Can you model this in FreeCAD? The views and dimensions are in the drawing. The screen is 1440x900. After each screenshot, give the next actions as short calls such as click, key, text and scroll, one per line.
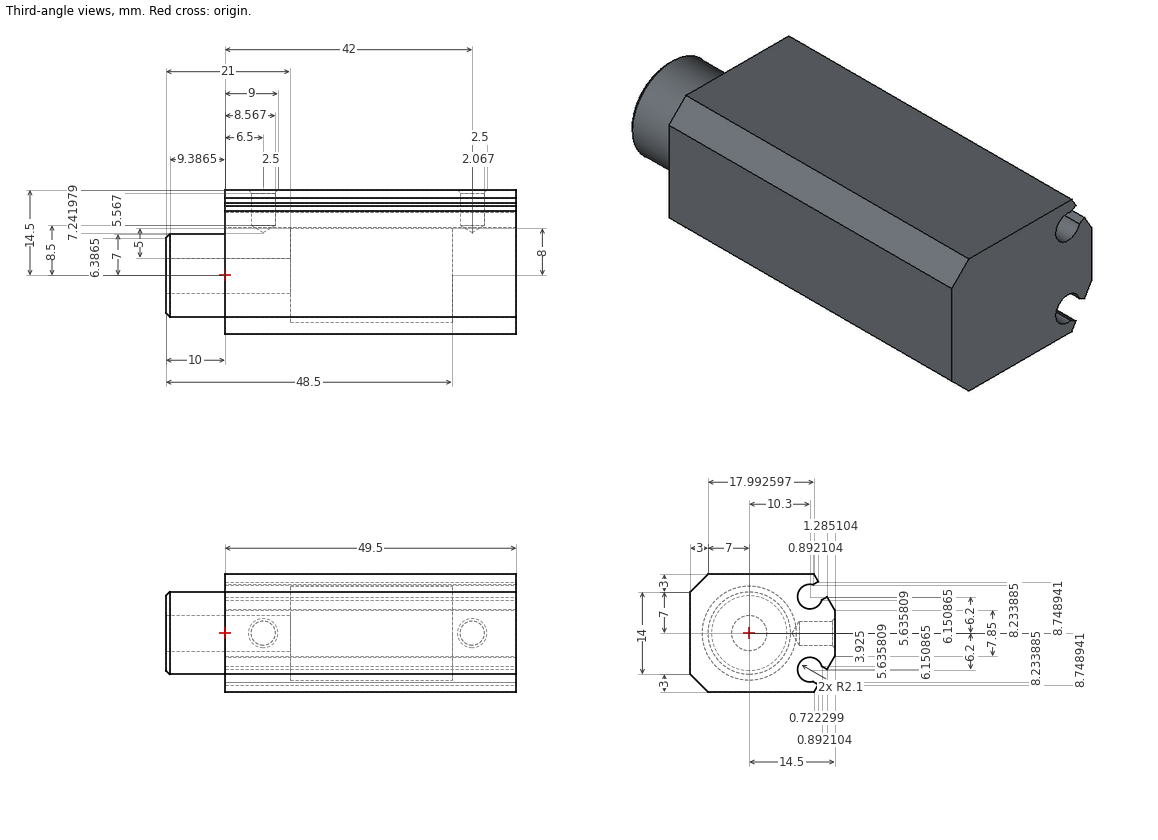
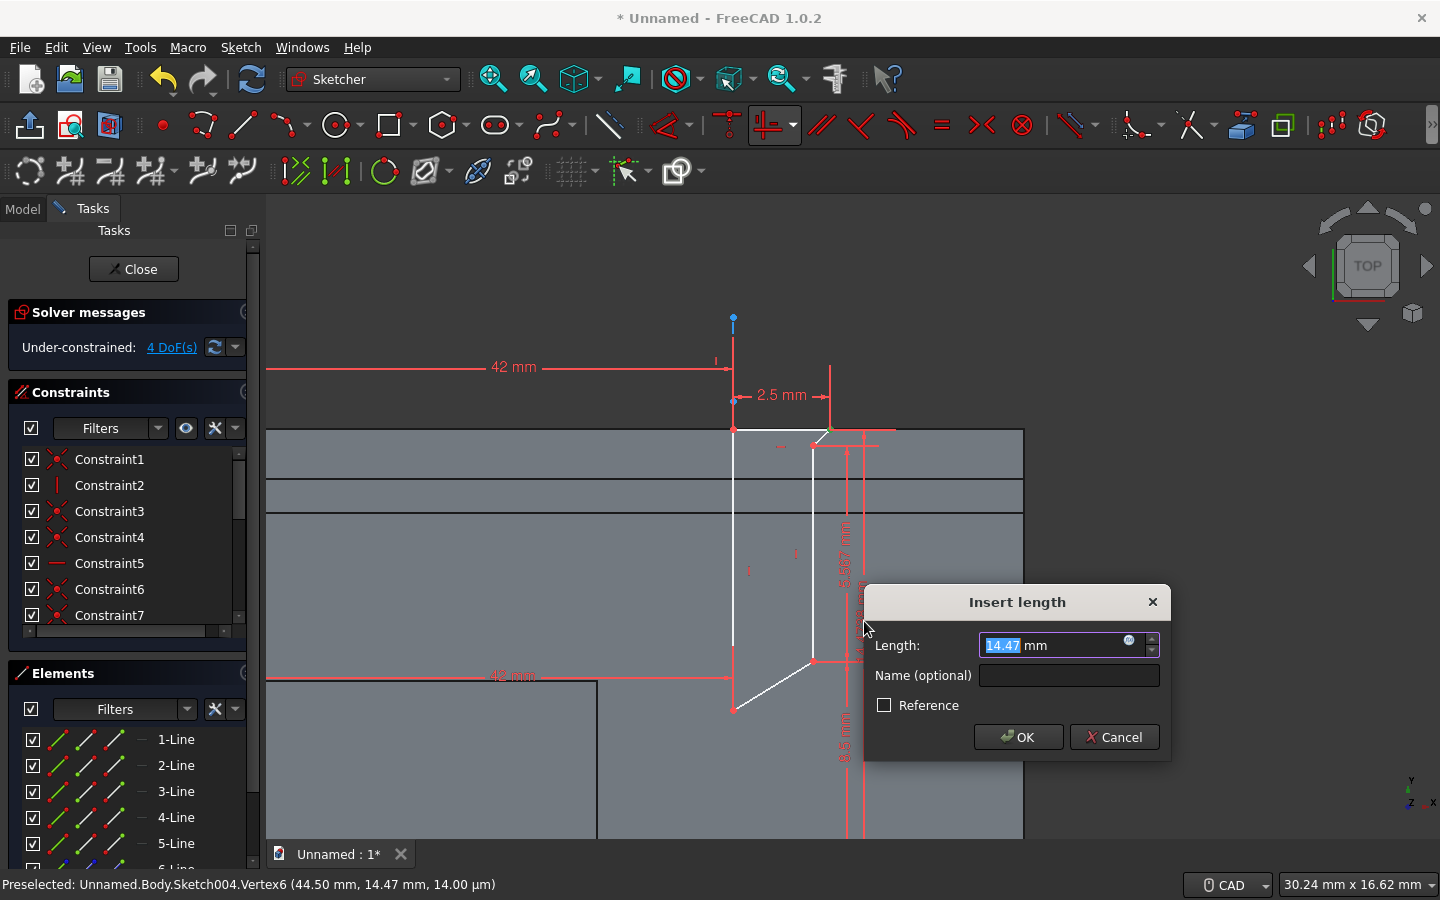
text(14.5)
key(Return)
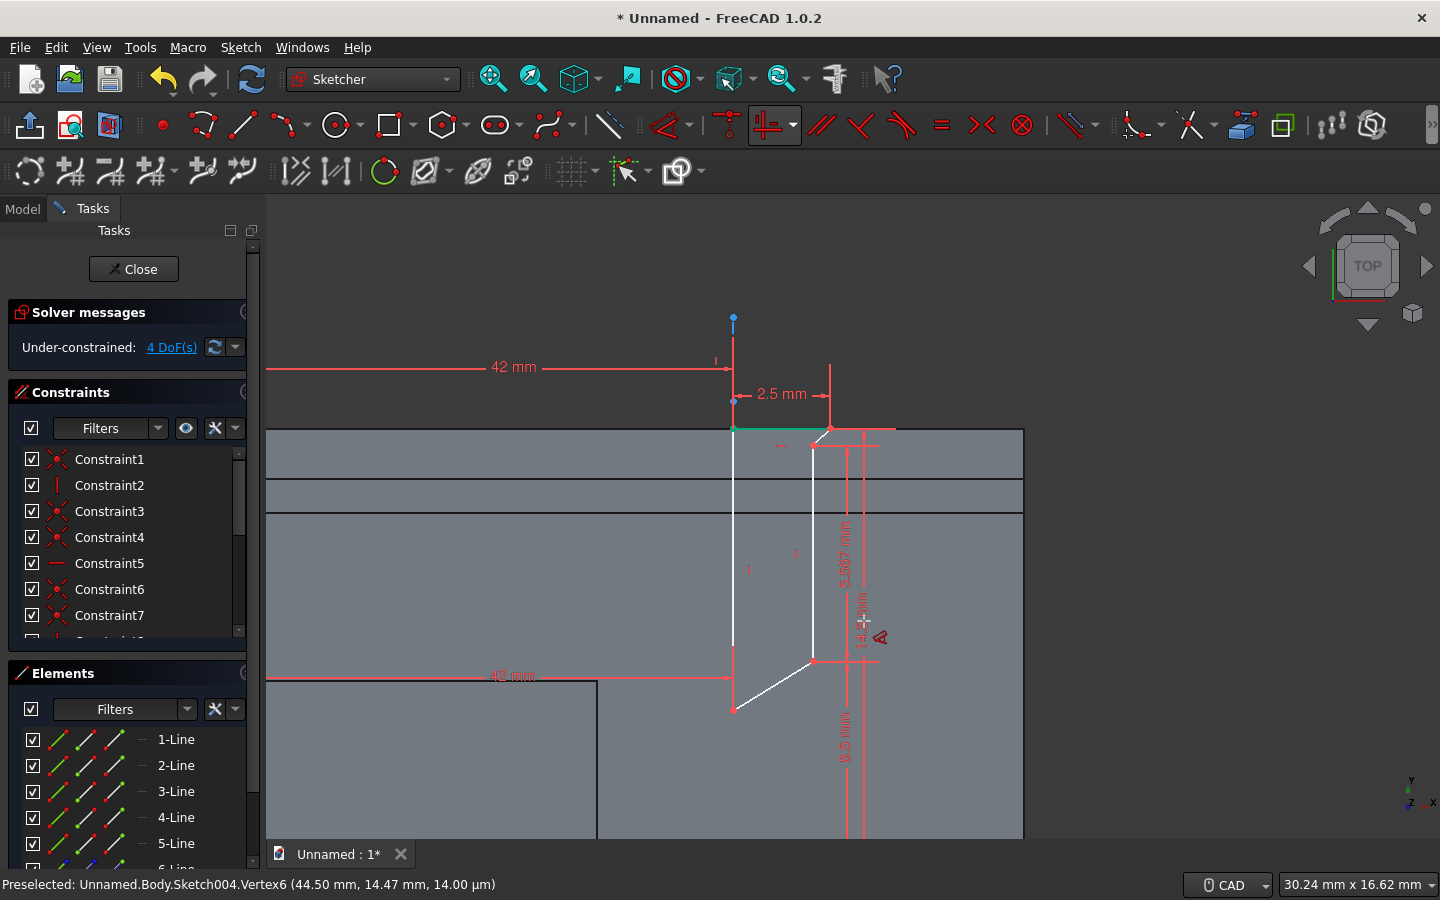
click(757, 696)
click(773, 745)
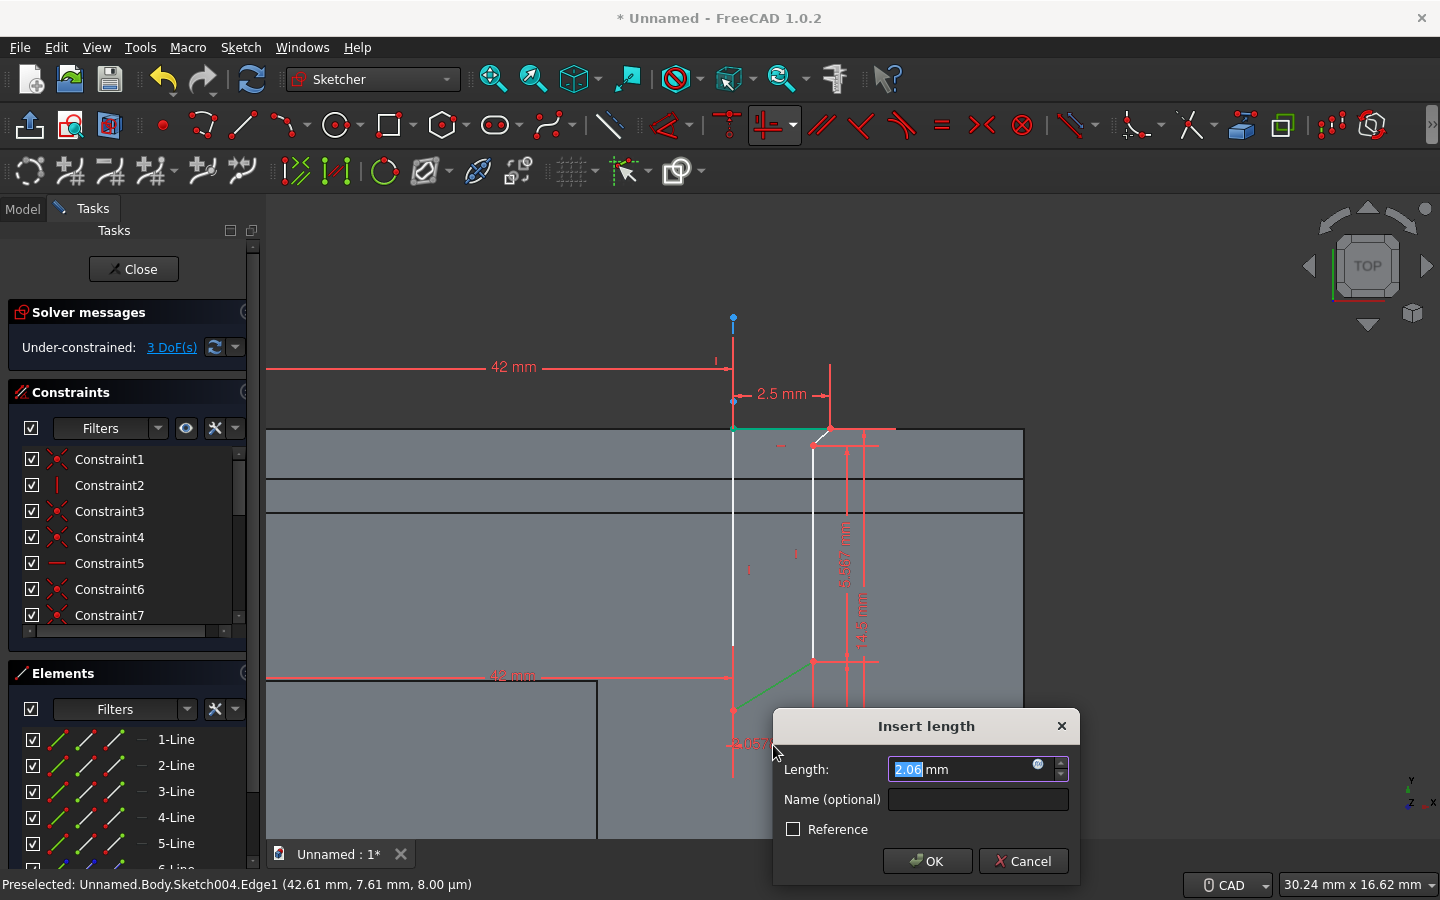
text(2.067)
key(Return)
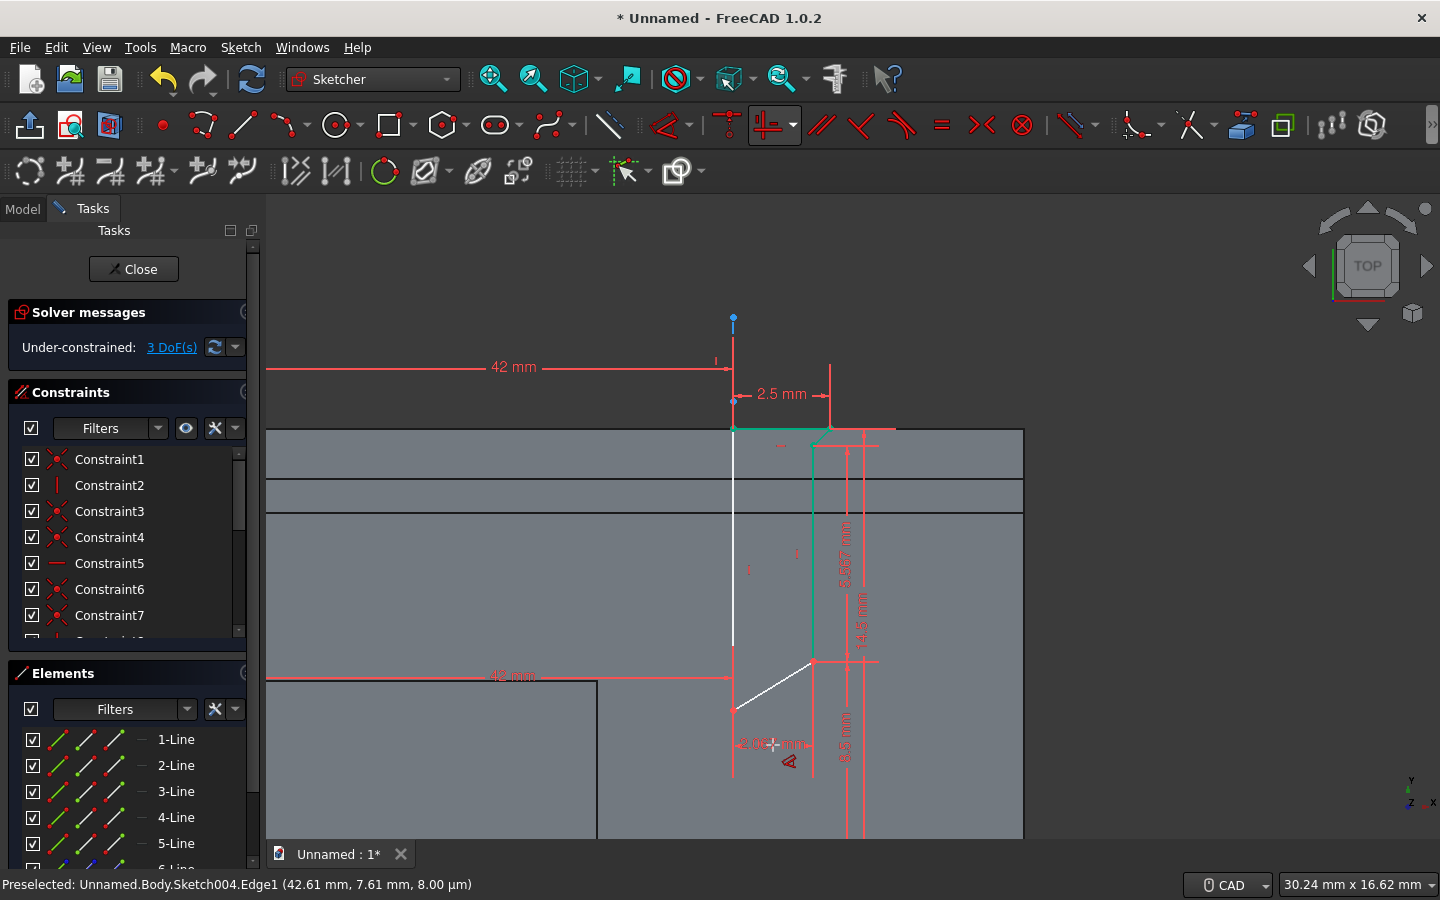
click(733, 514)
click(699, 570)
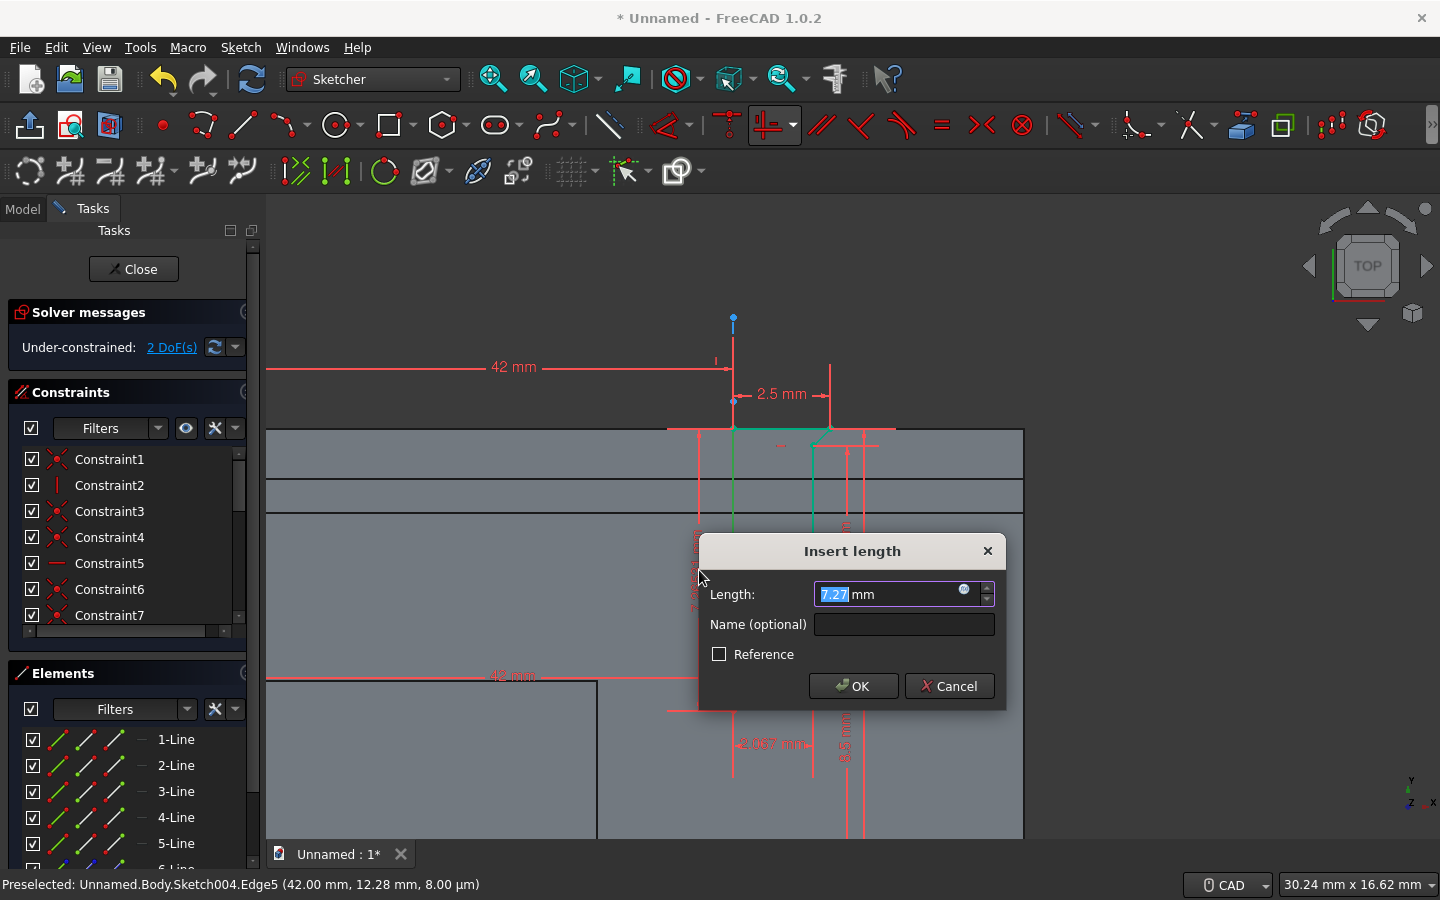
text(7.241979)
key(Return)
key(Escape)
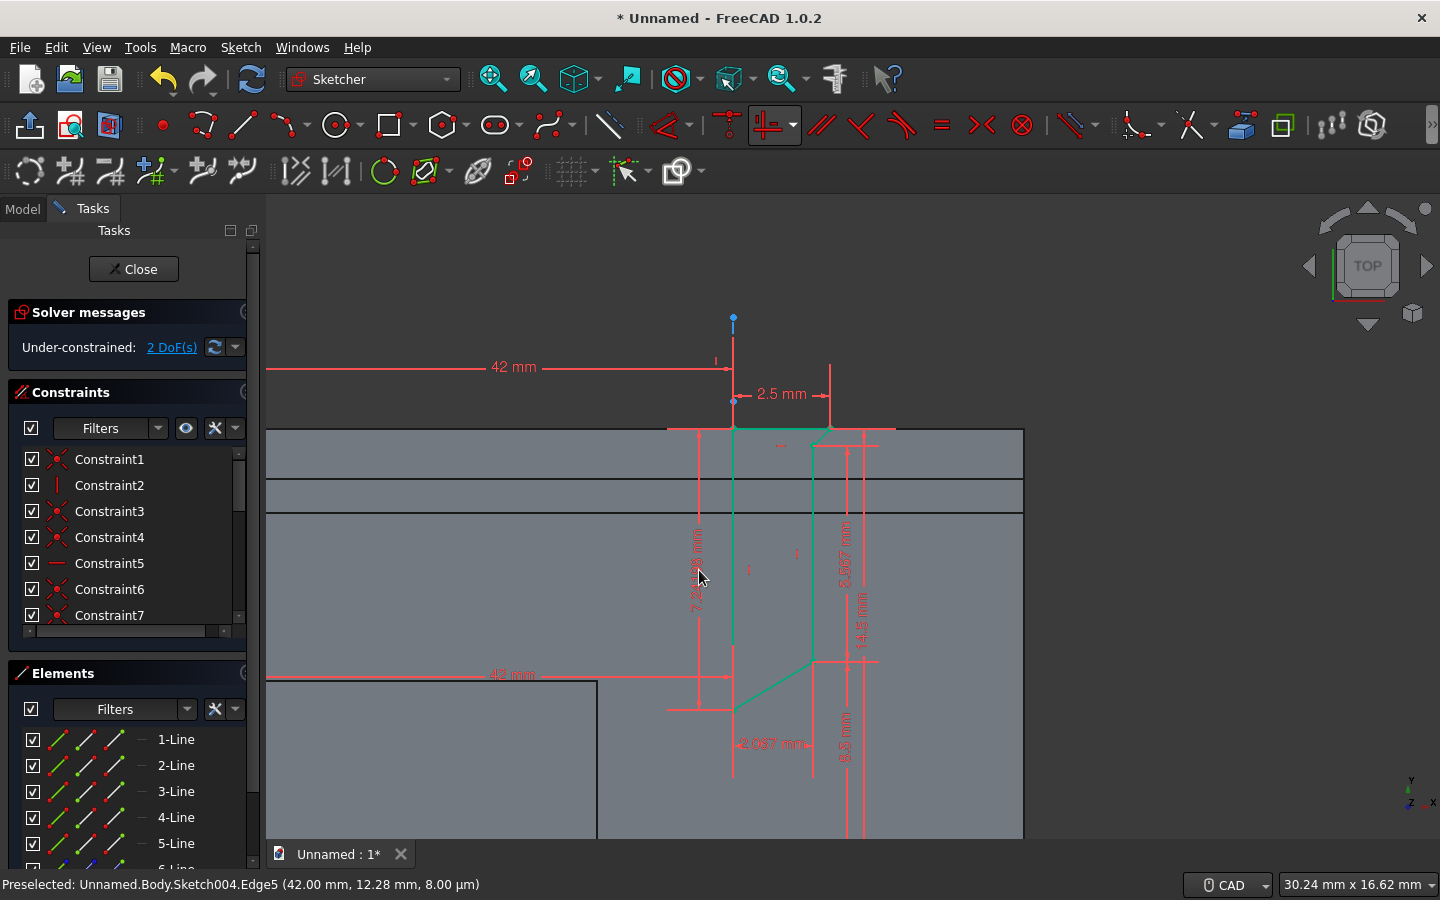
click(134, 269)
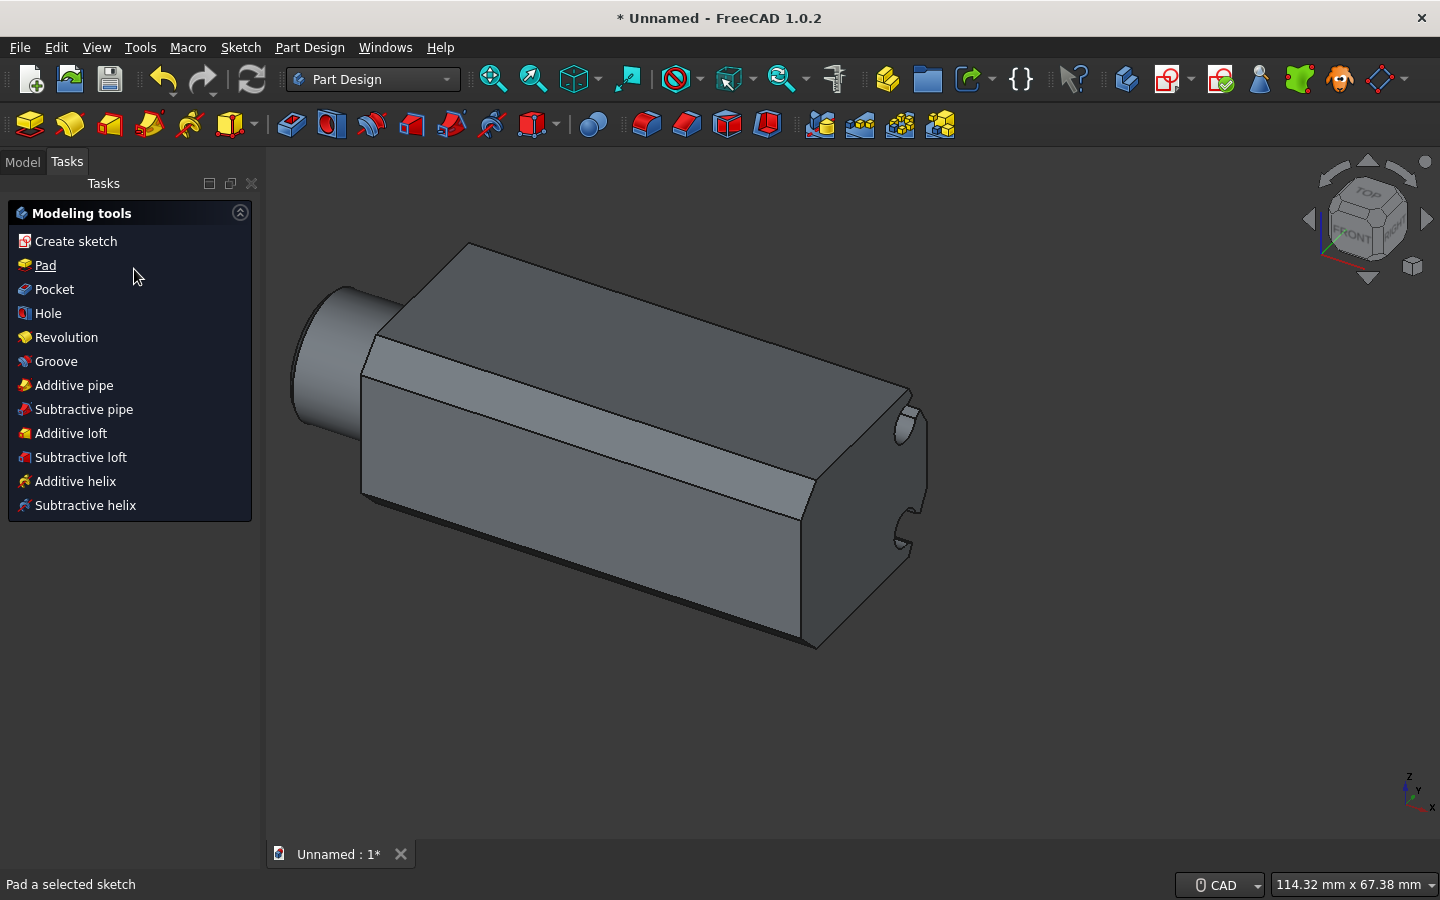
click(372, 124)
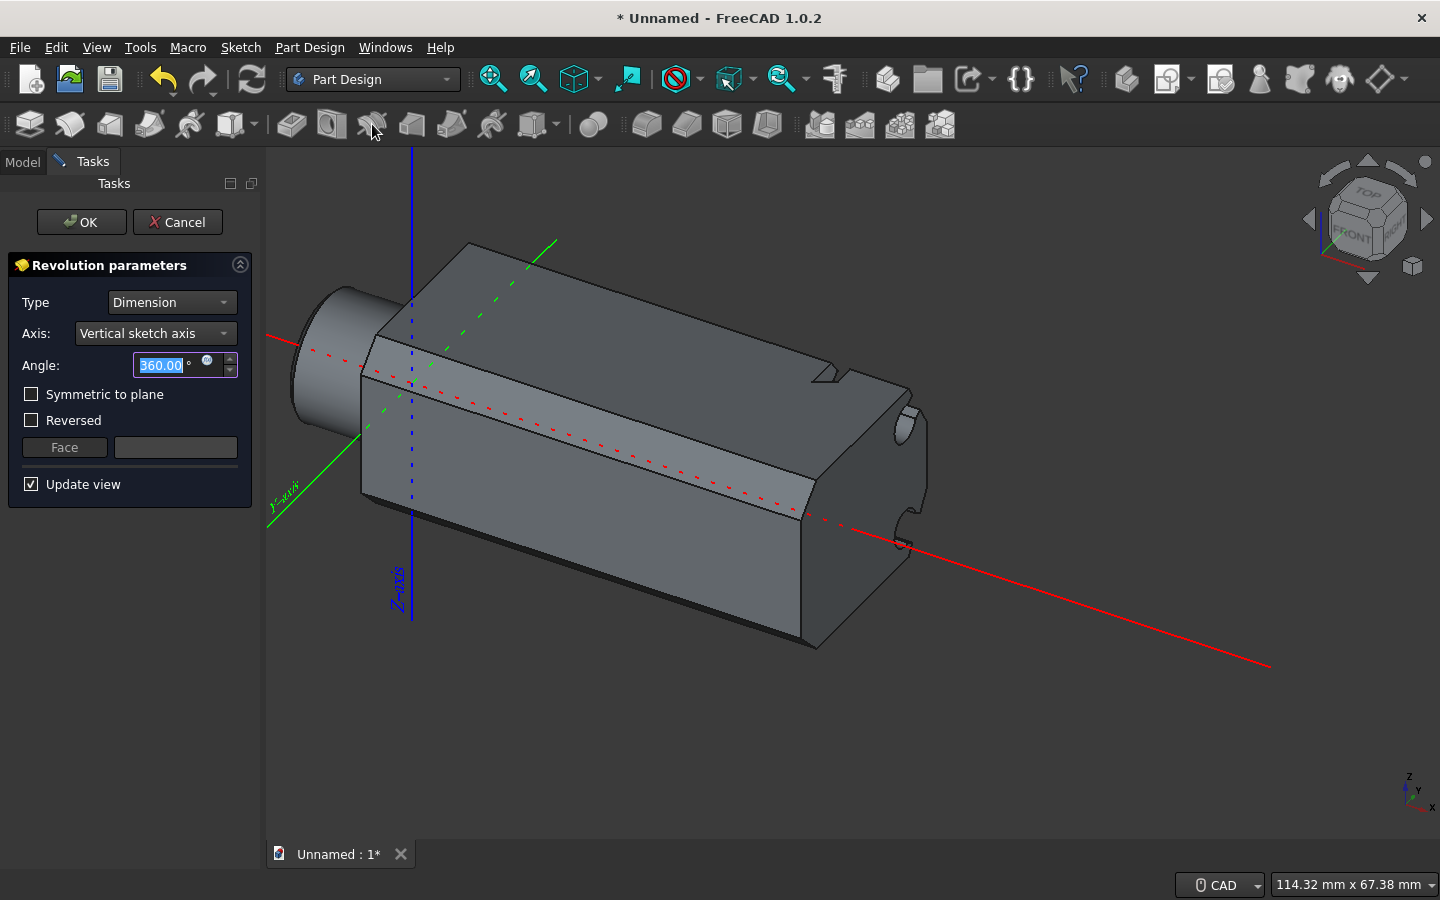
click(156, 334)